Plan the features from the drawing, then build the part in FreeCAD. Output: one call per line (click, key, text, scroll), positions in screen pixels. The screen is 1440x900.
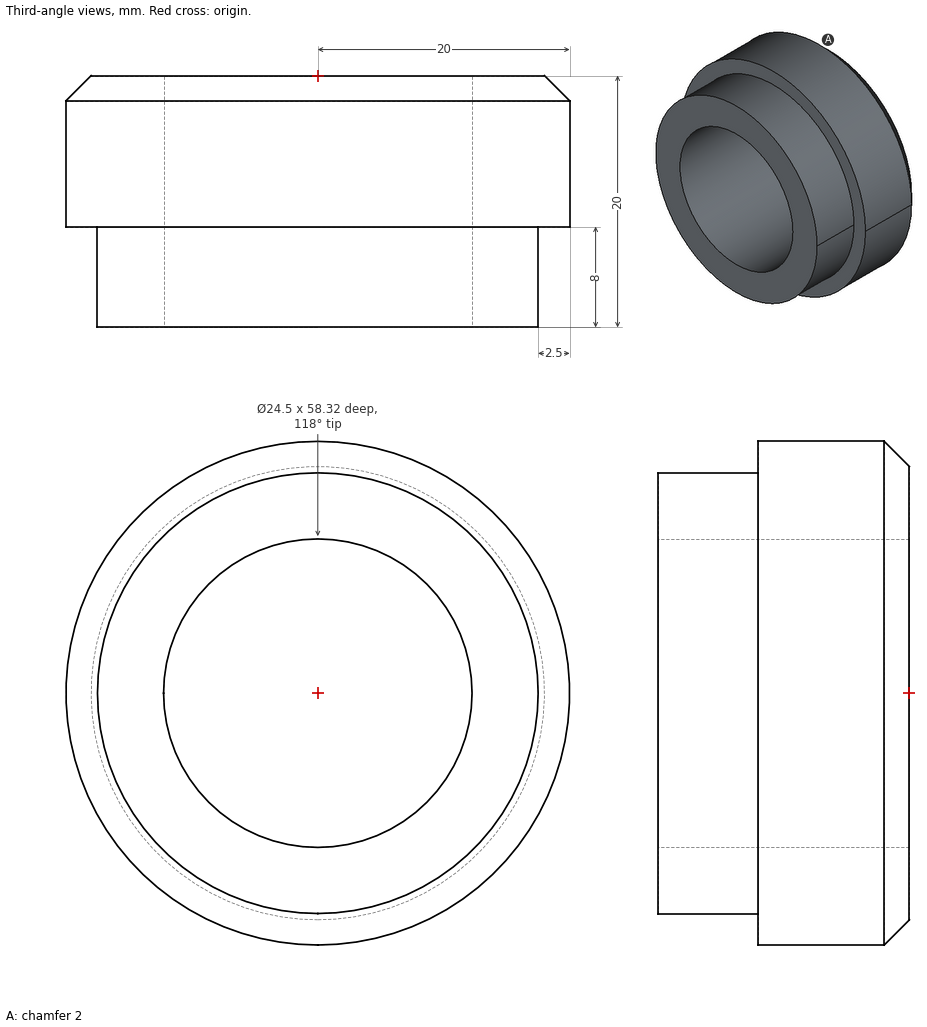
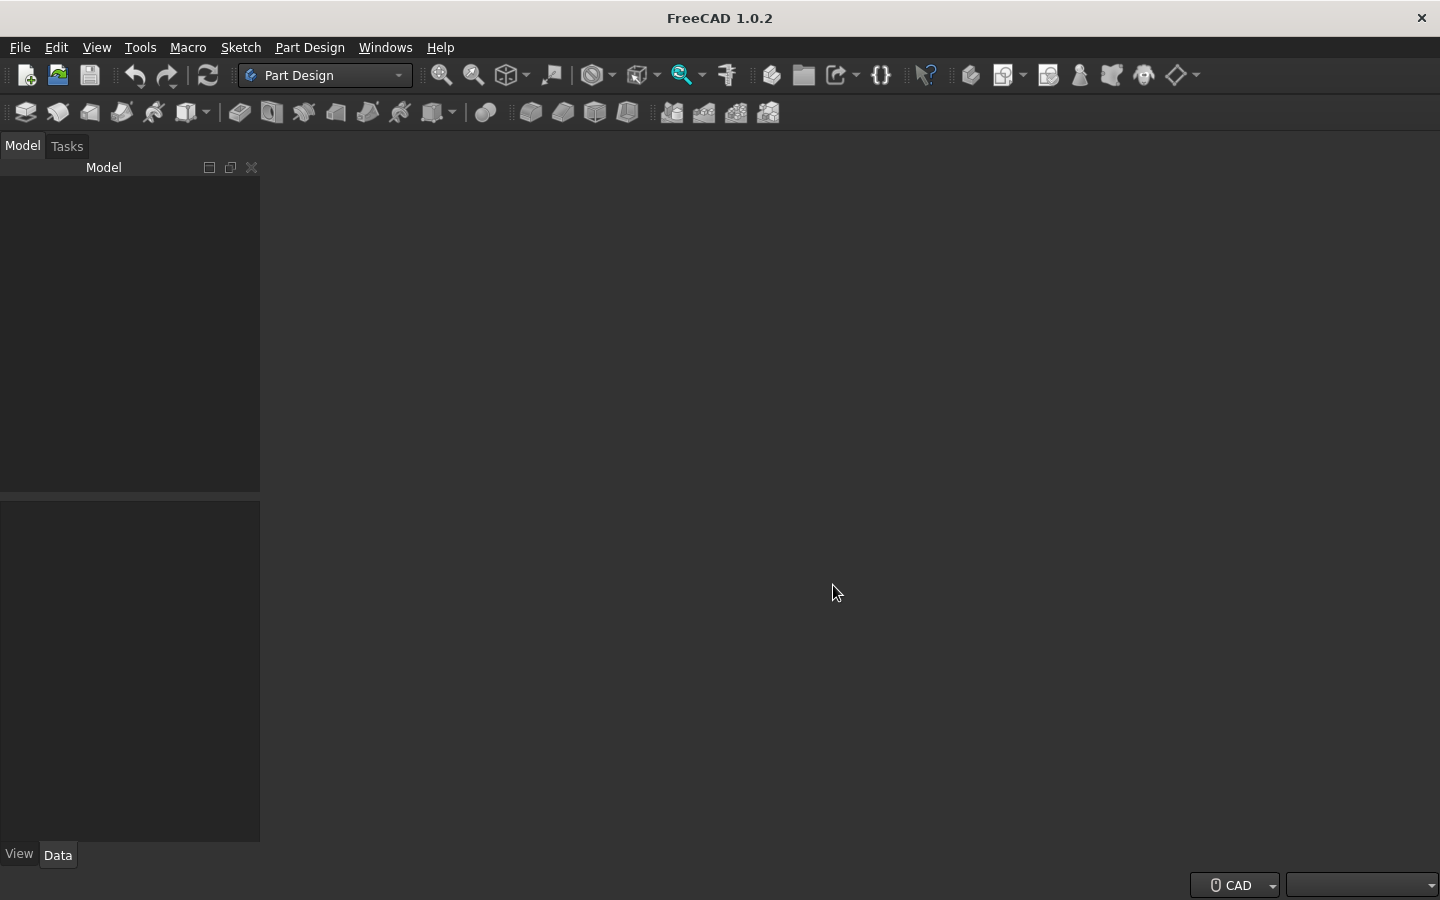
click(26, 76)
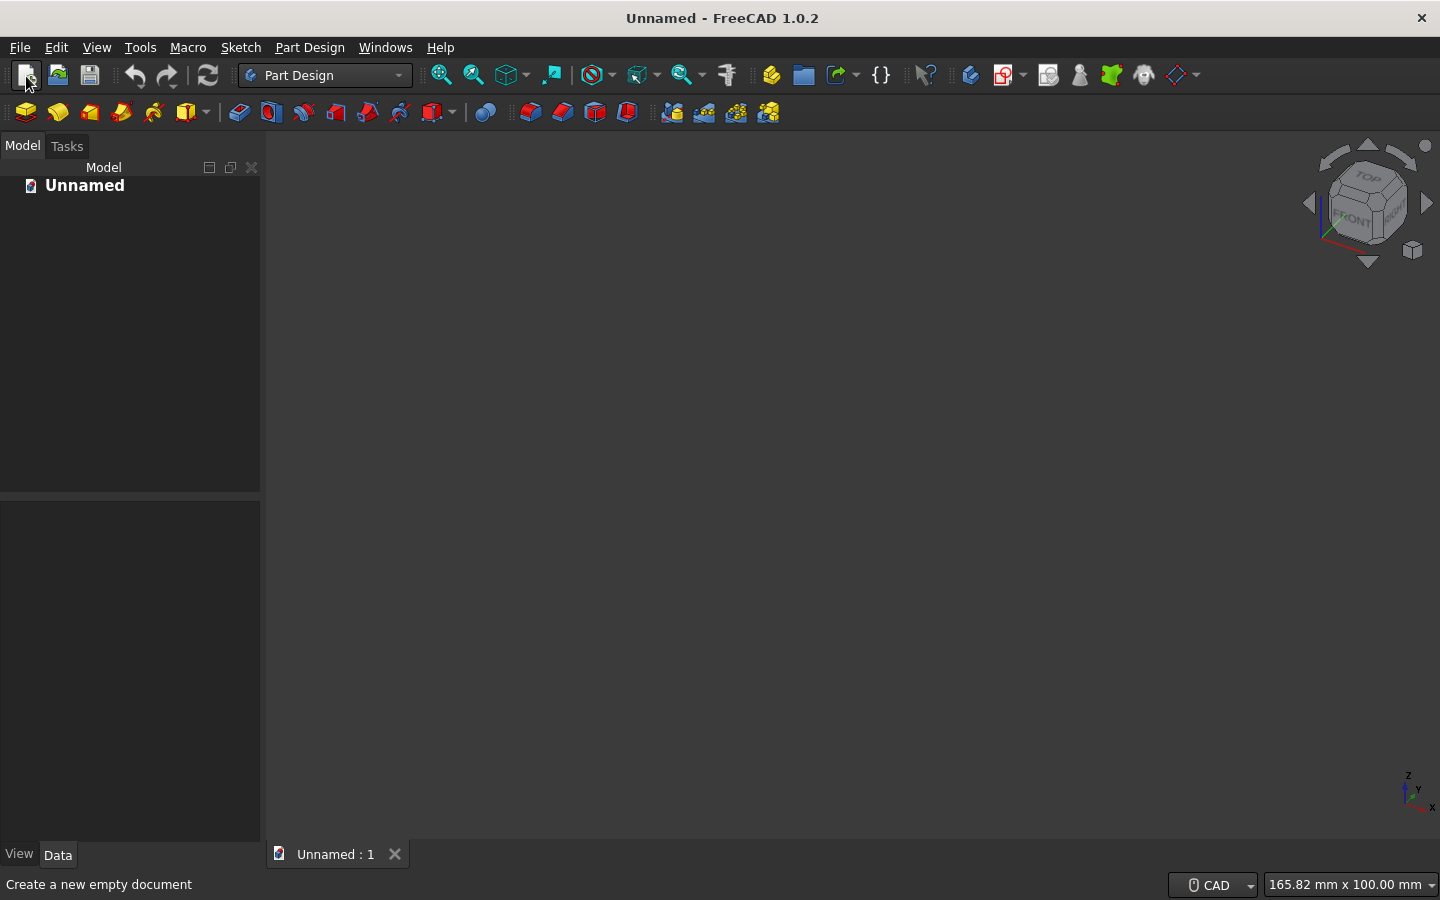
click(1004, 76)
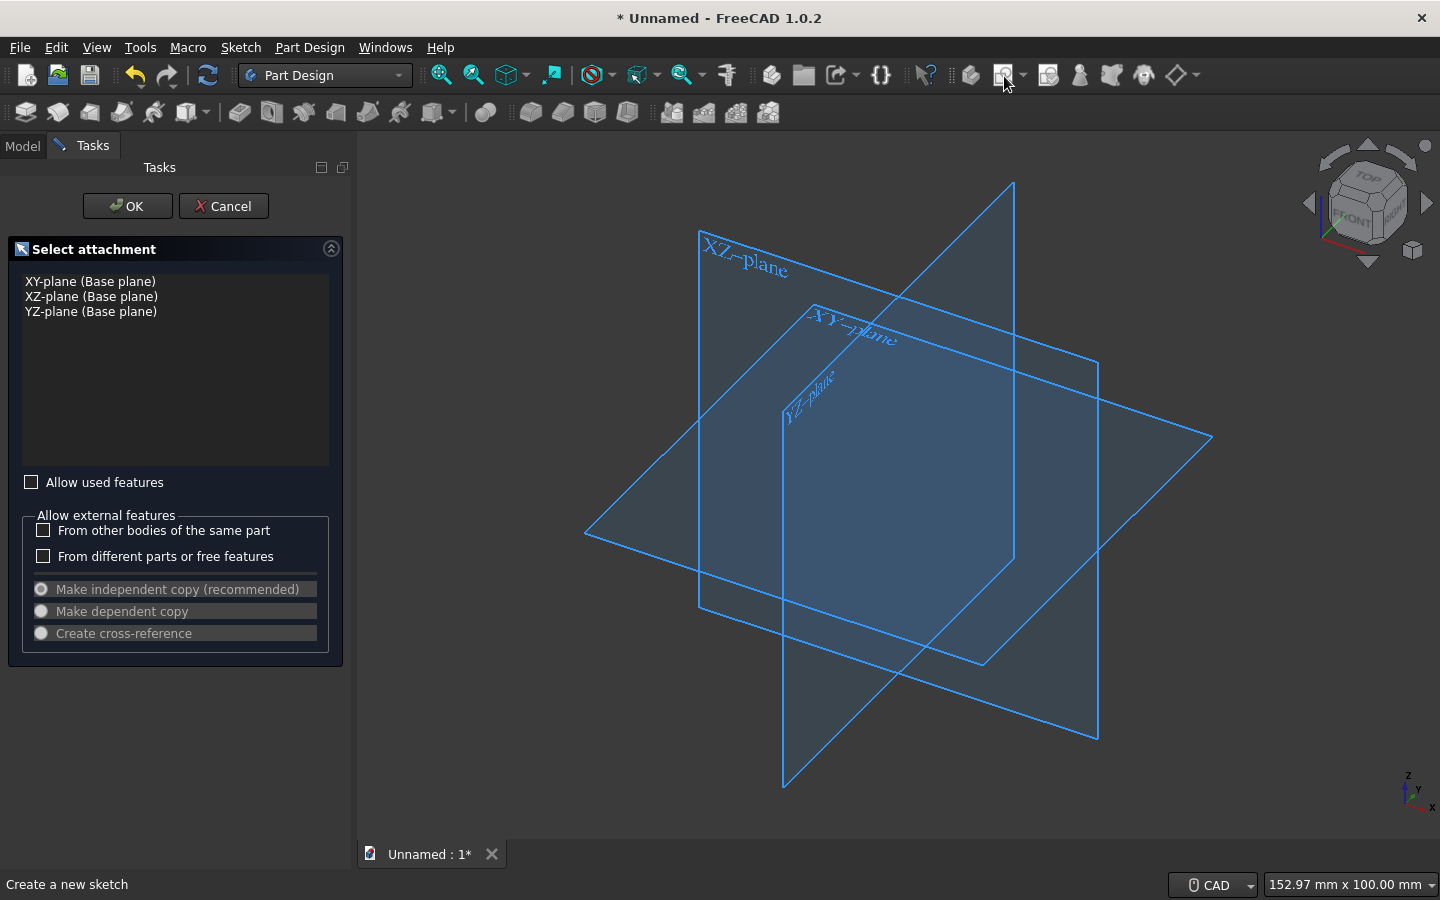
click(82, 282)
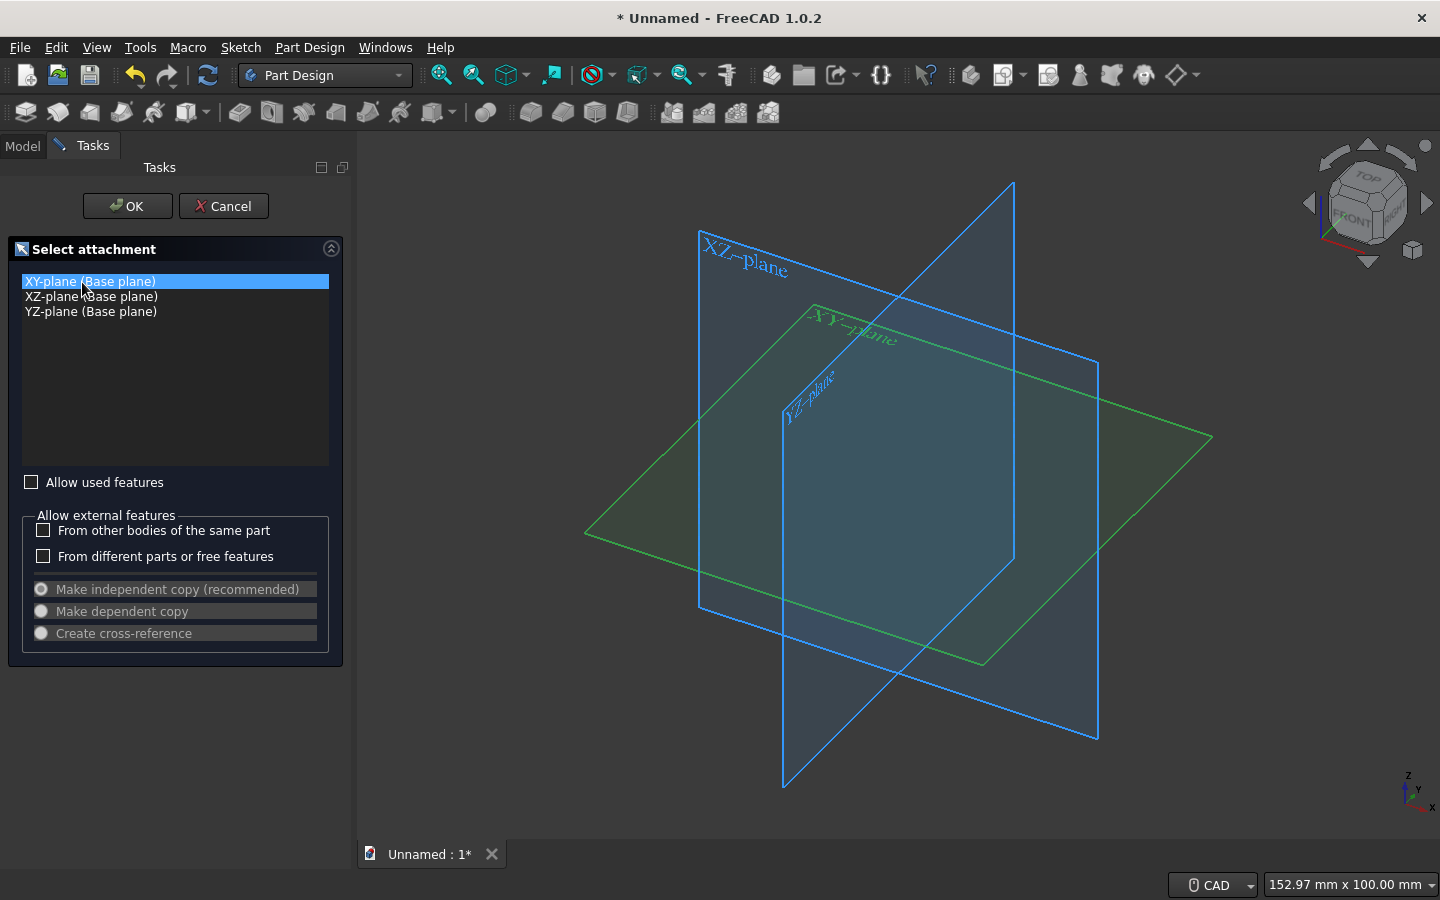
click(128, 206)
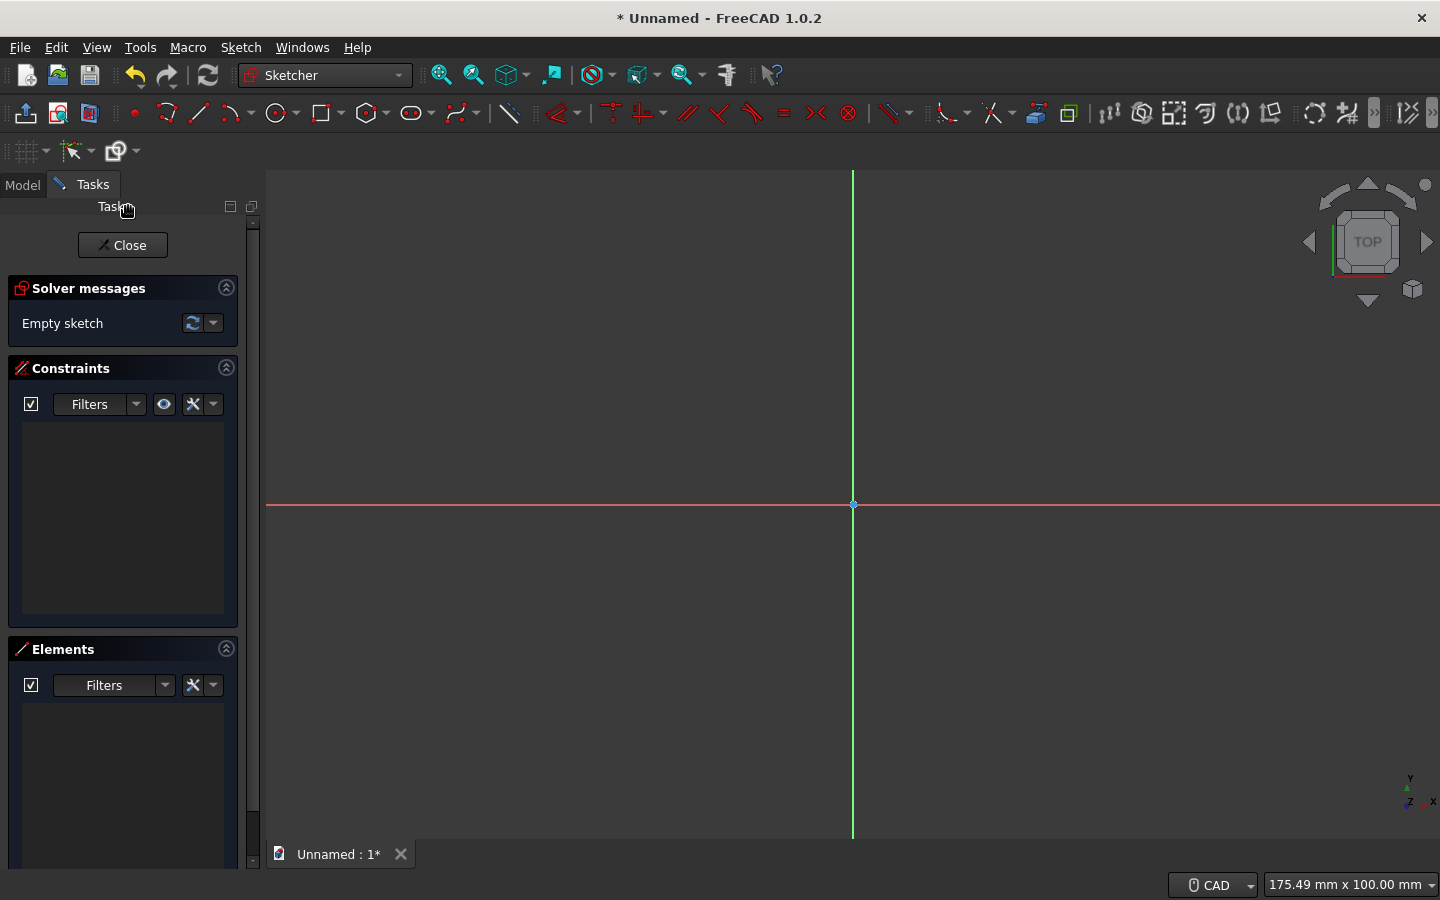
scroll(978, 600, up, 6)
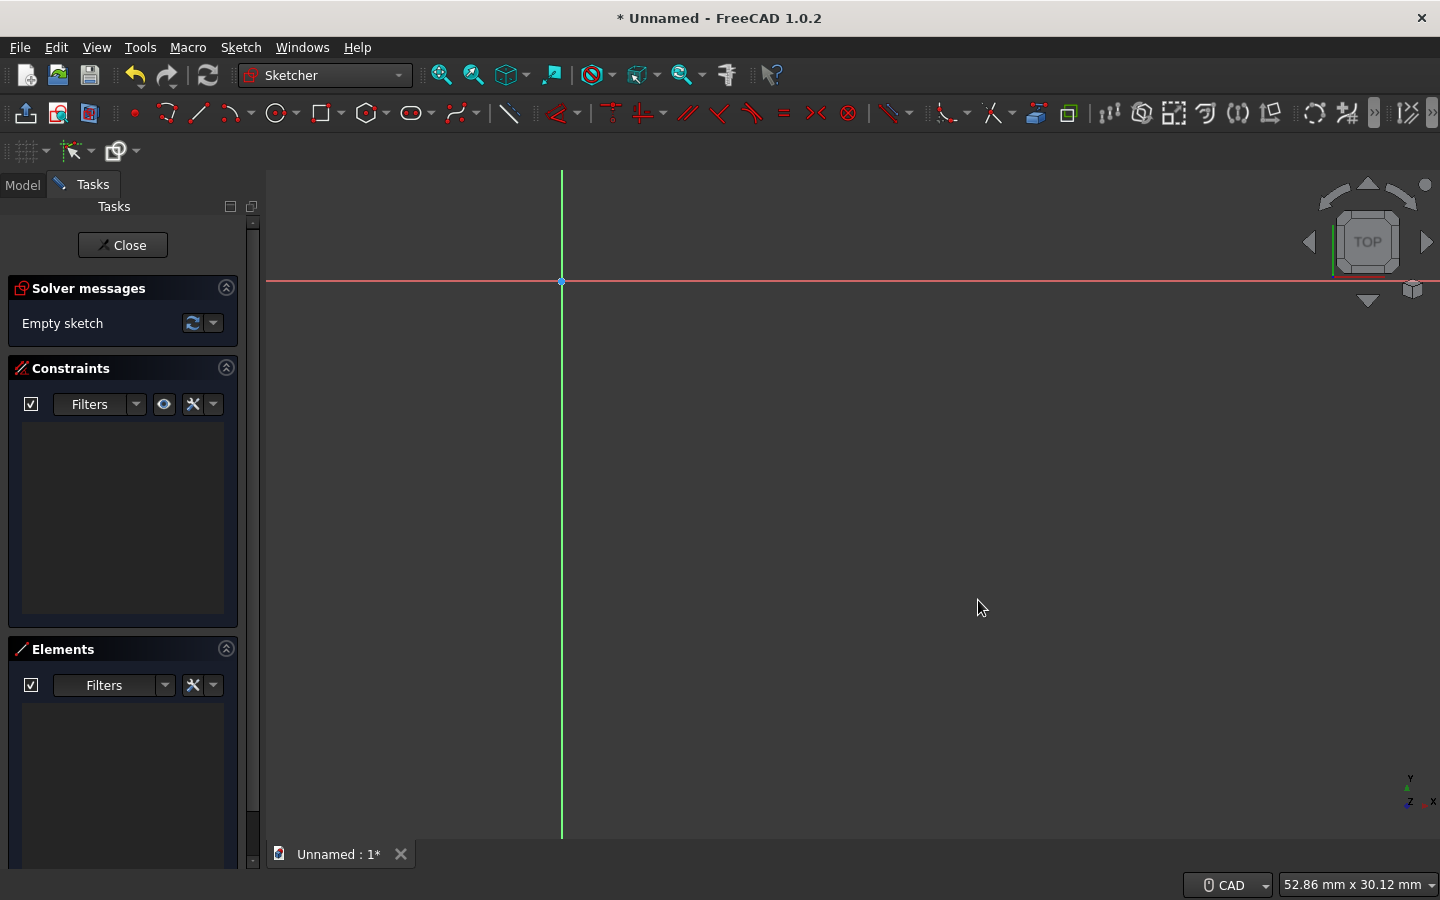
click(168, 114)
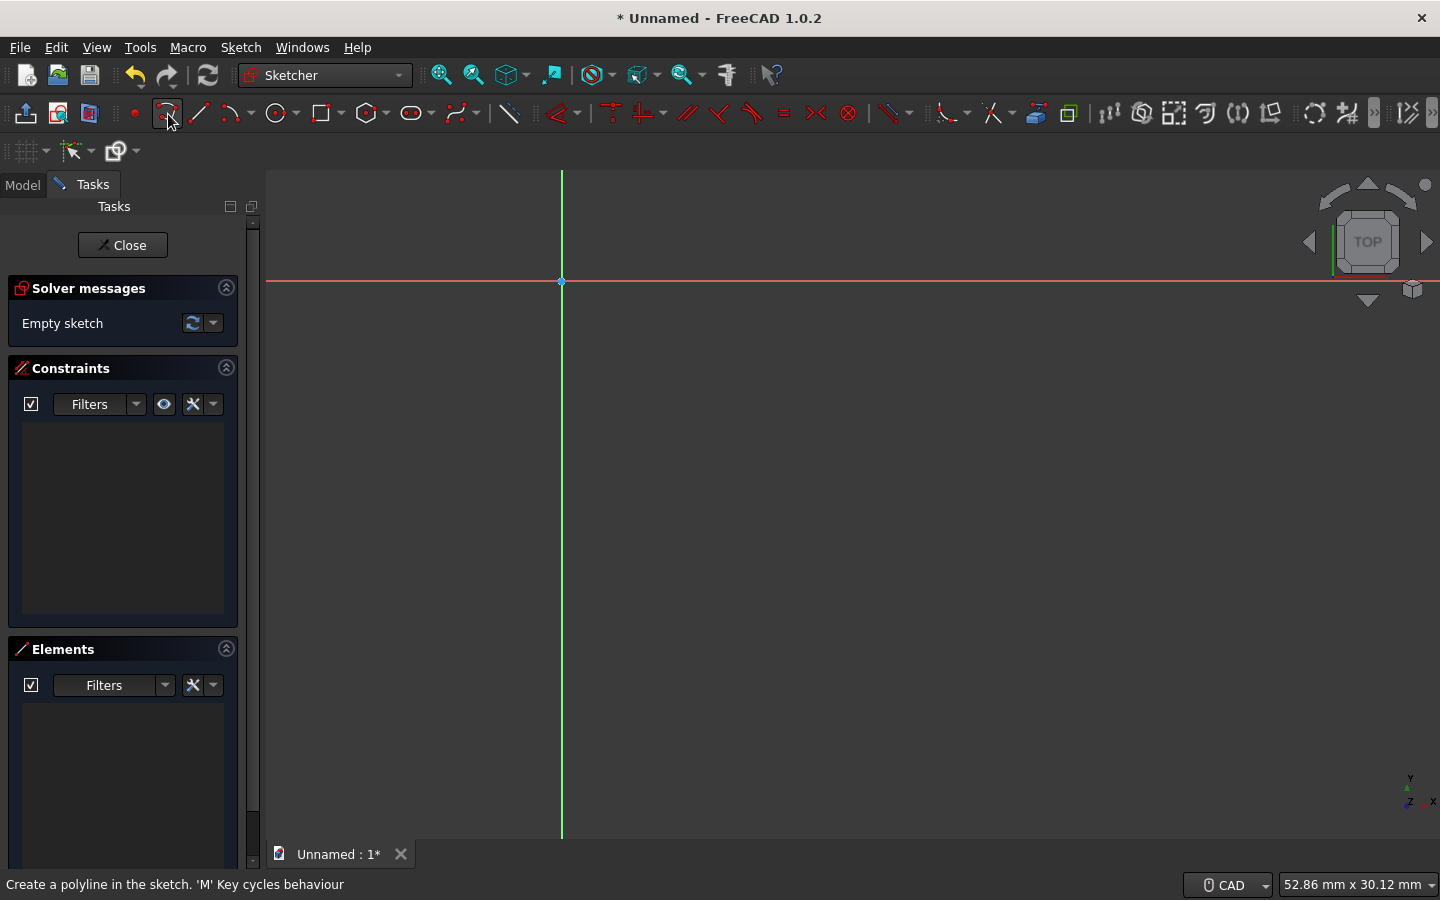
click(562, 281)
click(571, 726)
click(950, 726)
click(950, 548)
click(1006, 548)
click(1006, 290)
click(562, 281)
key(Escape)
key(Escape)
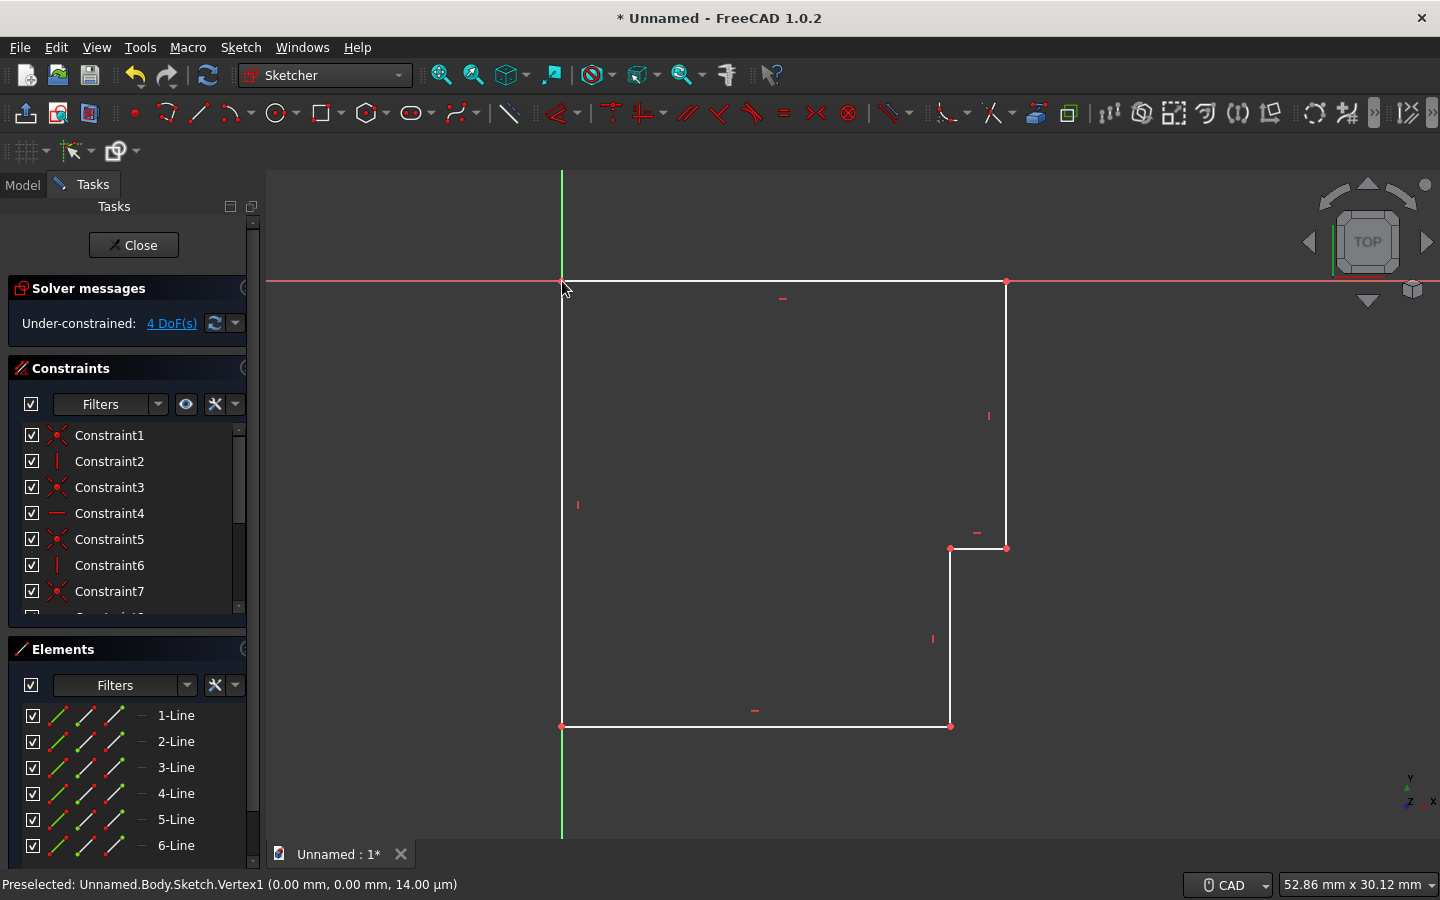
click(950, 674)